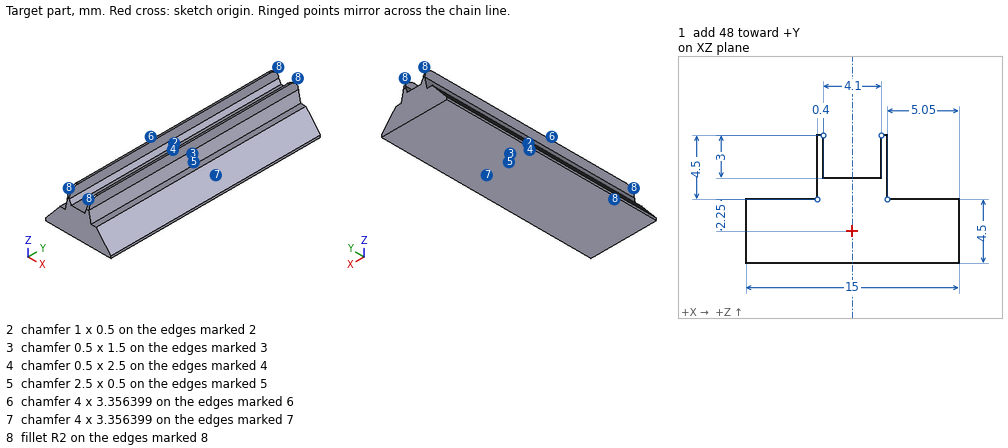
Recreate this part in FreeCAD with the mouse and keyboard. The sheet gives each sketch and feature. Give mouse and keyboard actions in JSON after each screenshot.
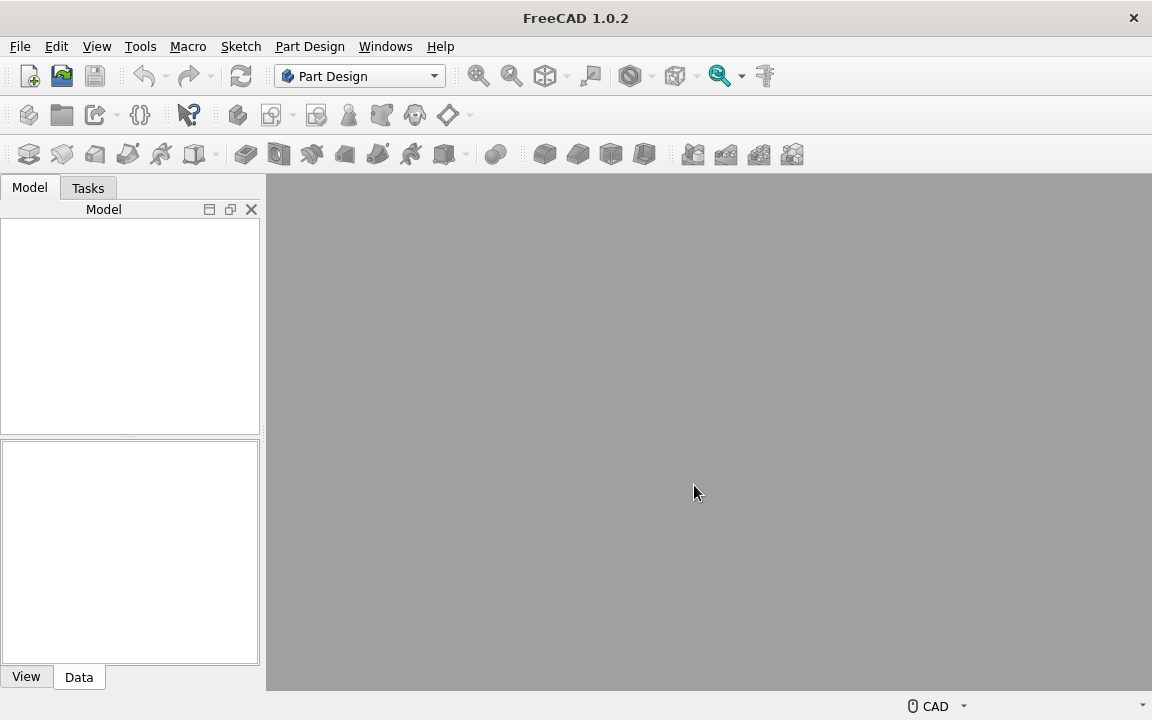
{"action": "left_click", "coordinate": [29, 76]}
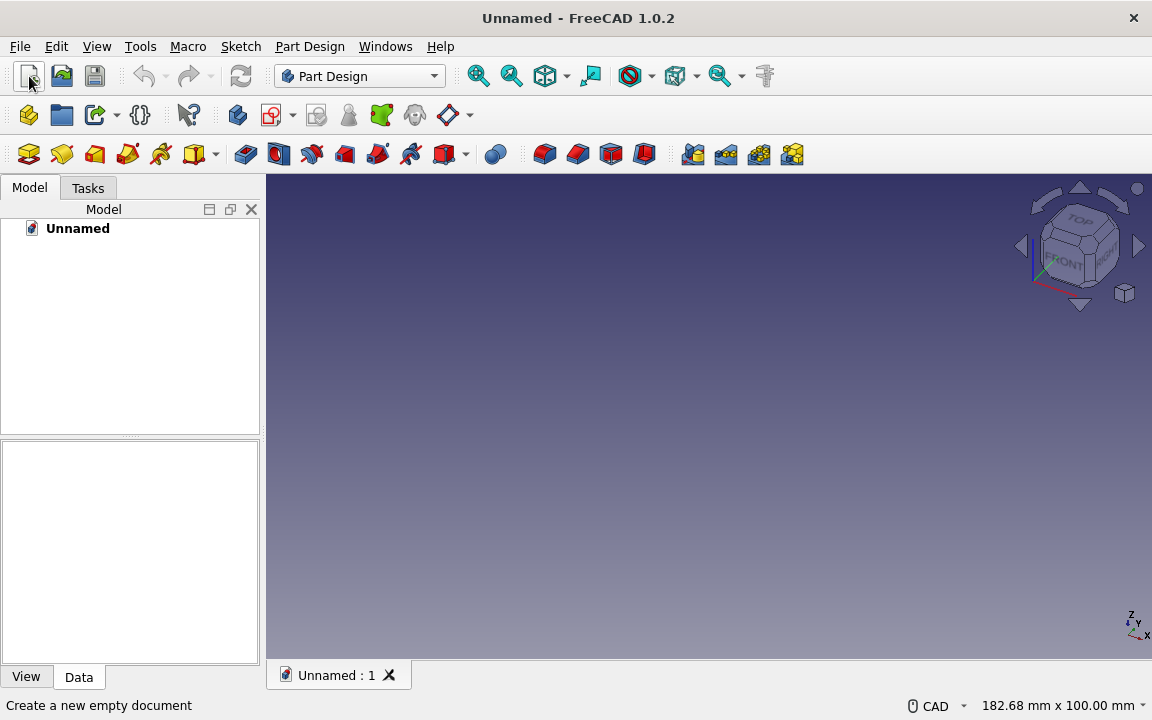
{"action": "left_click", "coordinate": [270, 116]}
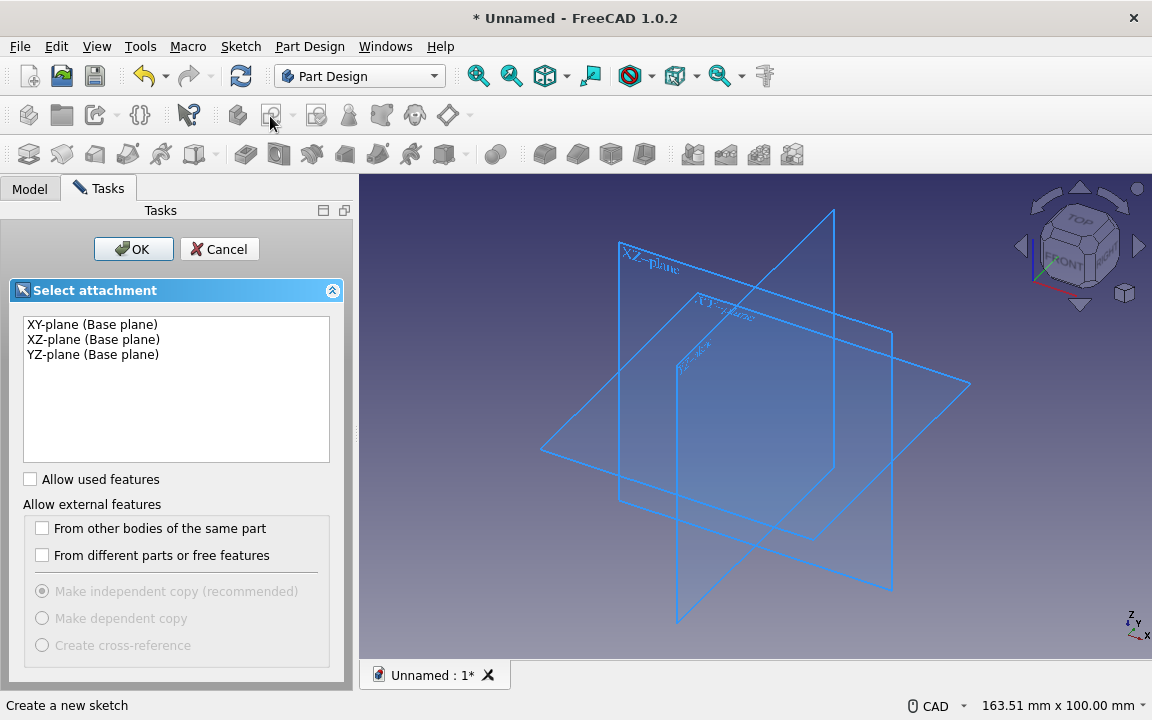
{"action": "left_click", "coordinate": [84, 340]}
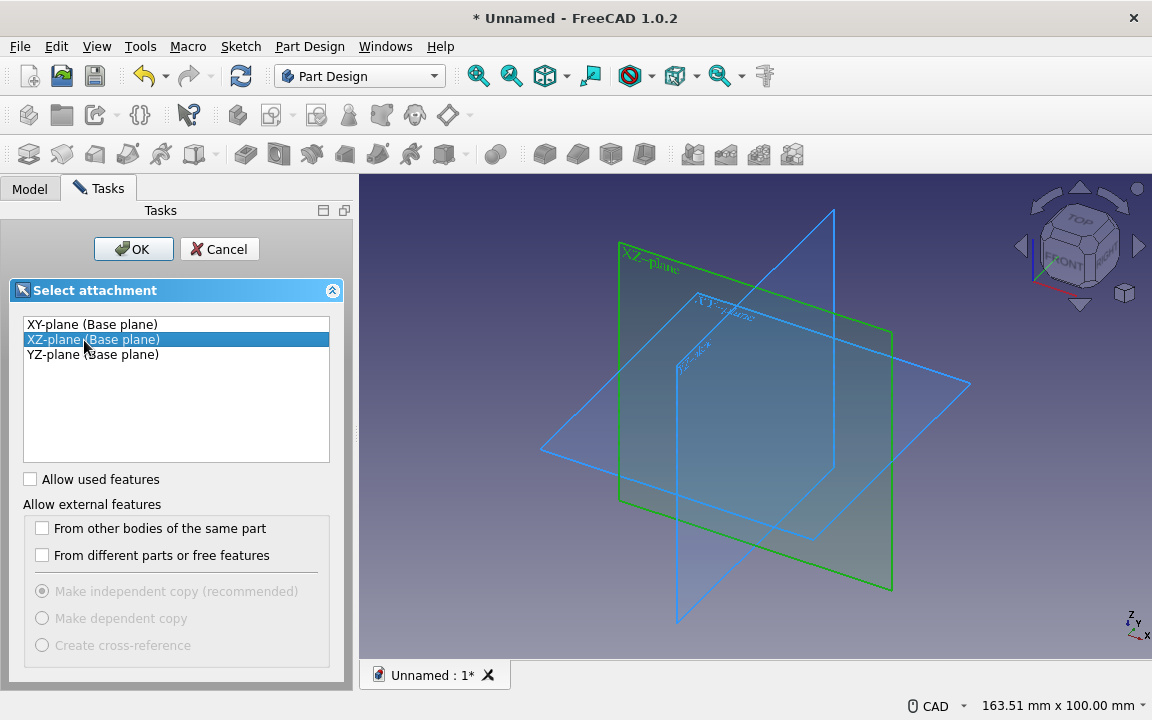
{"action": "left_click", "coordinate": [134, 249]}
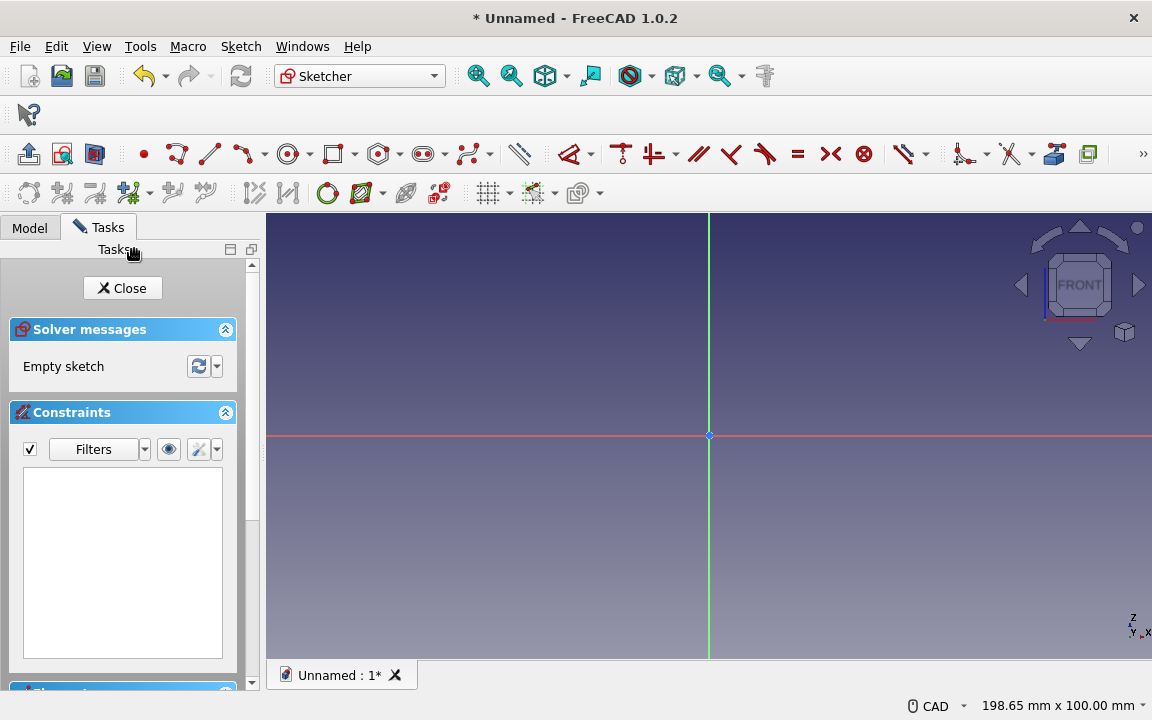
{"action": "scroll", "coordinate": [720, 424], "scroll_direction": "up", "scroll_amount": 10}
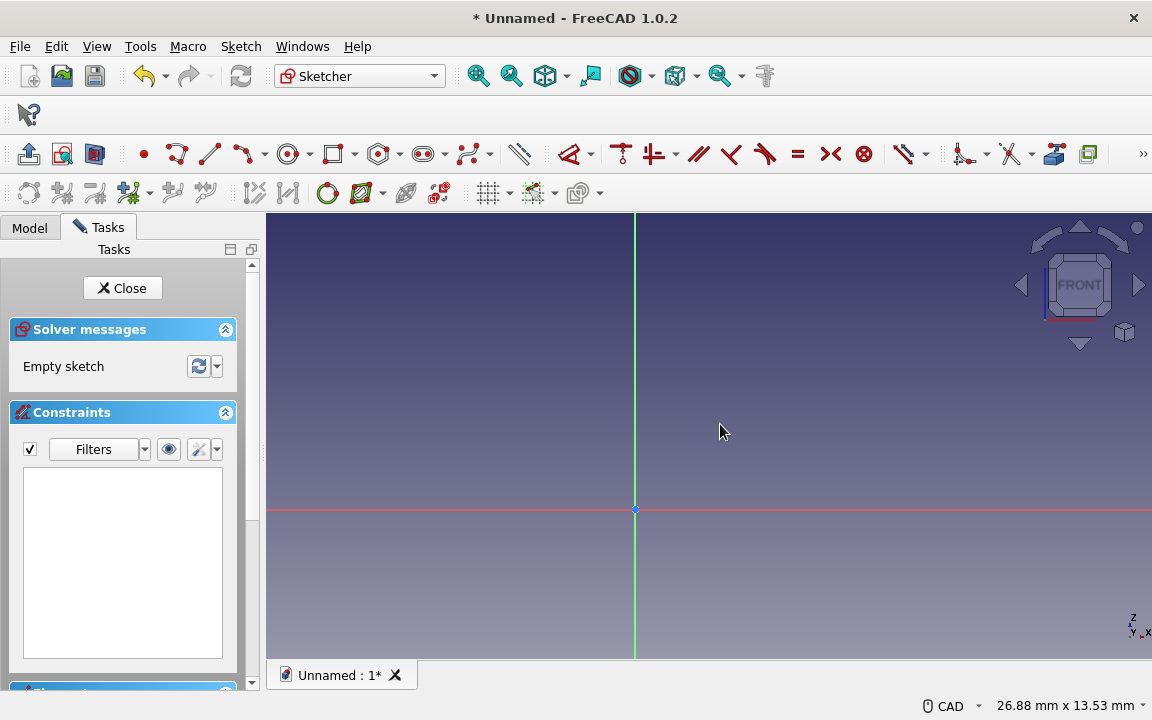
{"action": "left_click", "coordinate": [177, 154]}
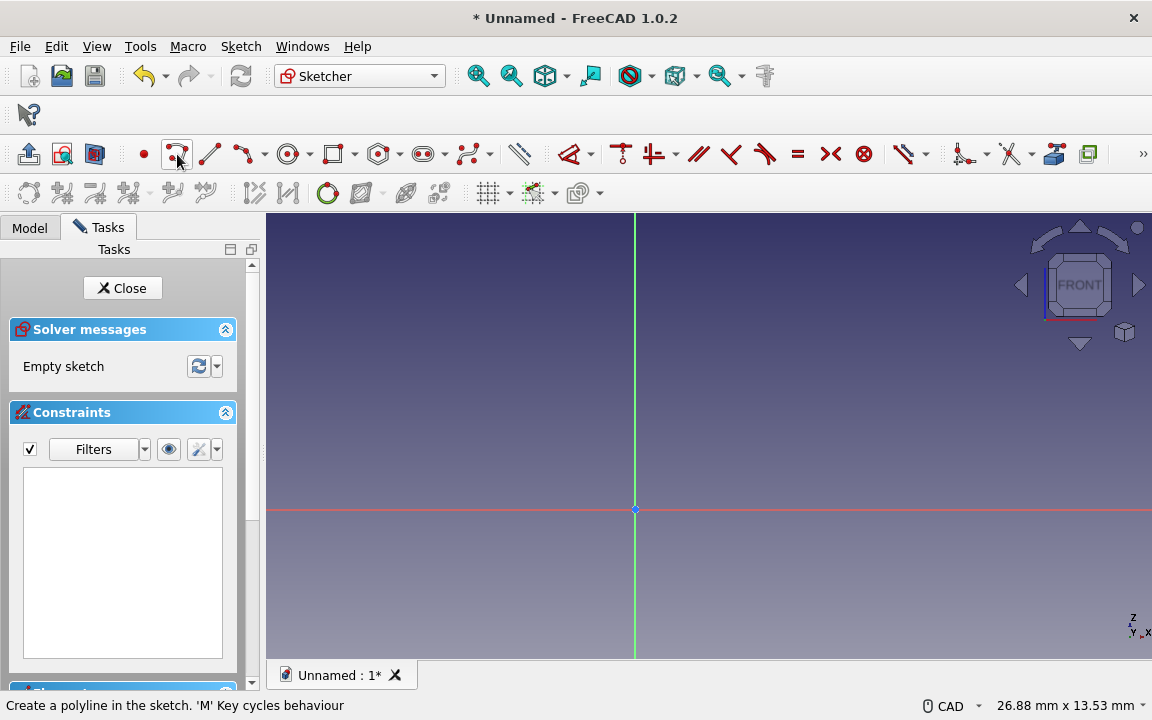
{"action": "left_click", "coordinate": [555, 435]}
{"action": "left_click", "coordinate": [555, 287]}
{"action": "left_click", "coordinate": [568, 287]}
{"action": "left_click", "coordinate": [568, 386]}
{"action": "left_click", "coordinate": [703, 386]}
{"action": "left_click", "coordinate": [703, 287]}
{"action": "left_click", "coordinate": [716, 287]}
{"action": "left_click", "coordinate": [716, 435]}
{"action": "left_click", "coordinate": [883, 435]}
{"action": "left_click", "coordinate": [883, 584]}
{"action": "left_click", "coordinate": [388, 584]}
{"action": "left_click", "coordinate": [388, 435]}
{"action": "left_click", "coordinate": [555, 436]}
{"action": "key", "text": "Escape"}
{"action": "key", "text": "Escape"}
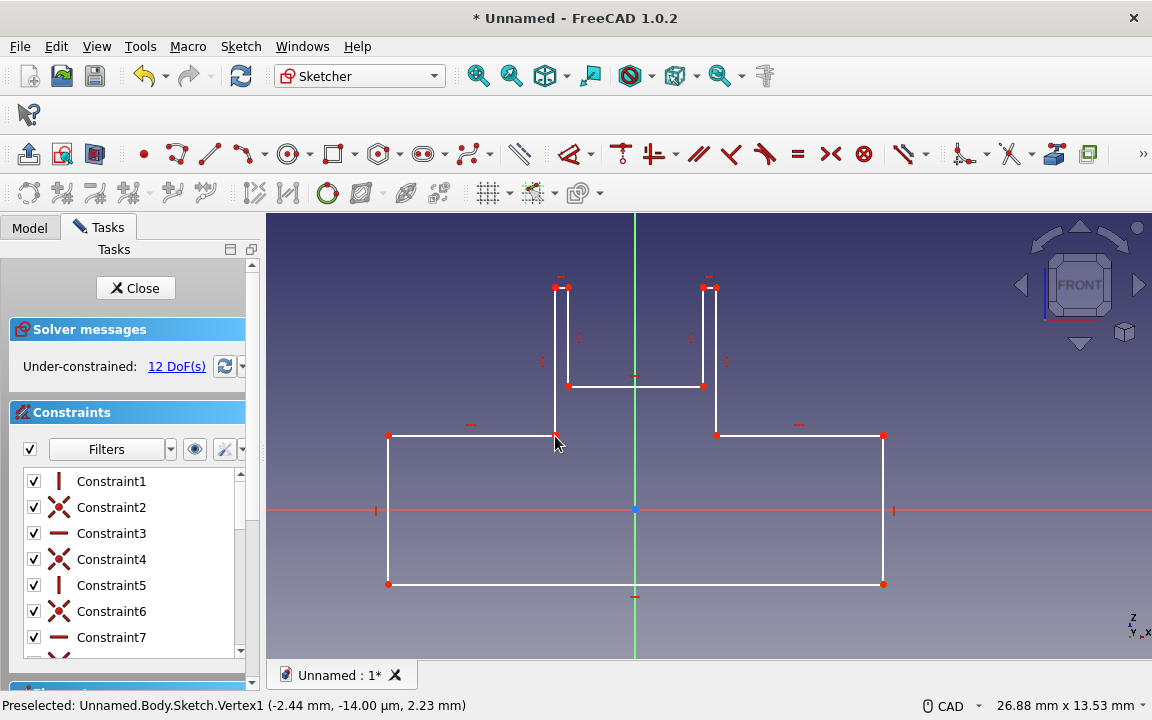
{"action": "left_click", "coordinate": [568, 288]}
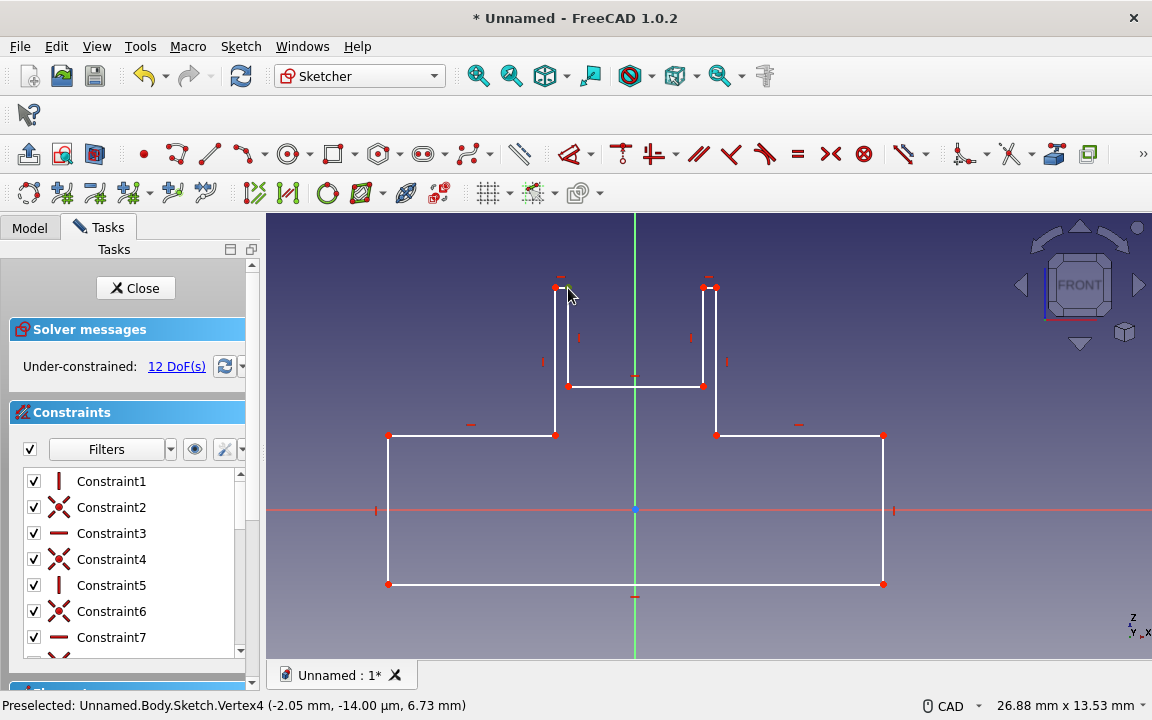
{"action": "left_click", "coordinate": [703, 288]}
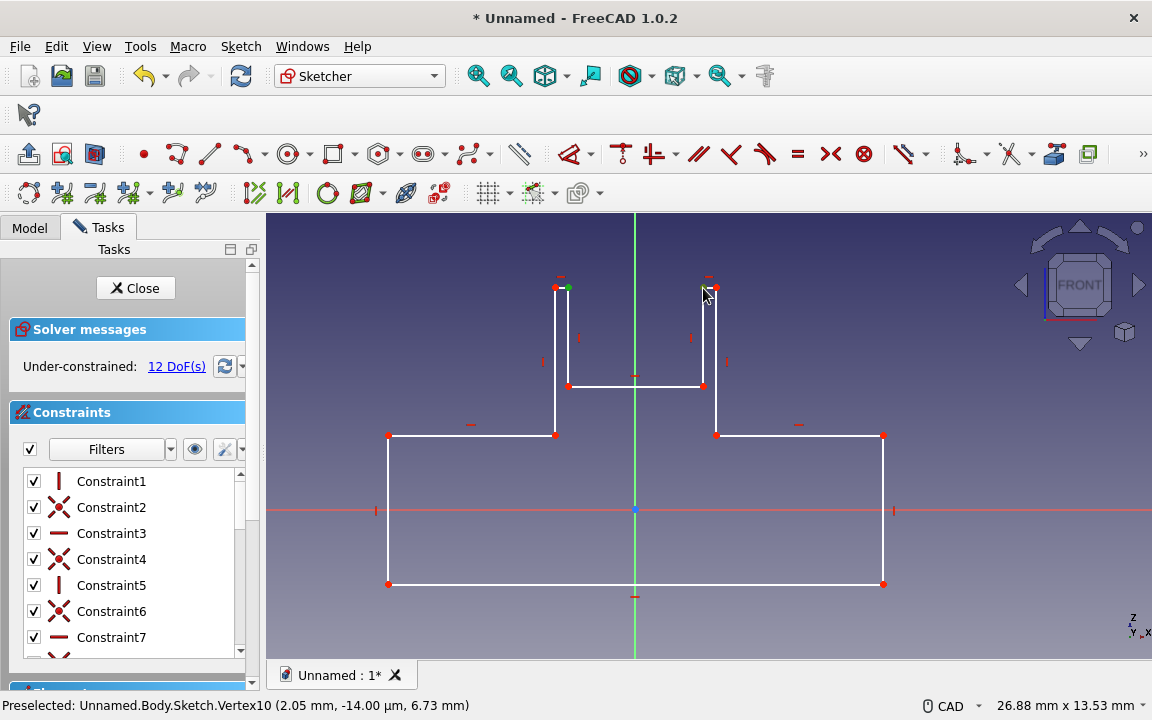
{"action": "left_click", "coordinate": [635, 547]}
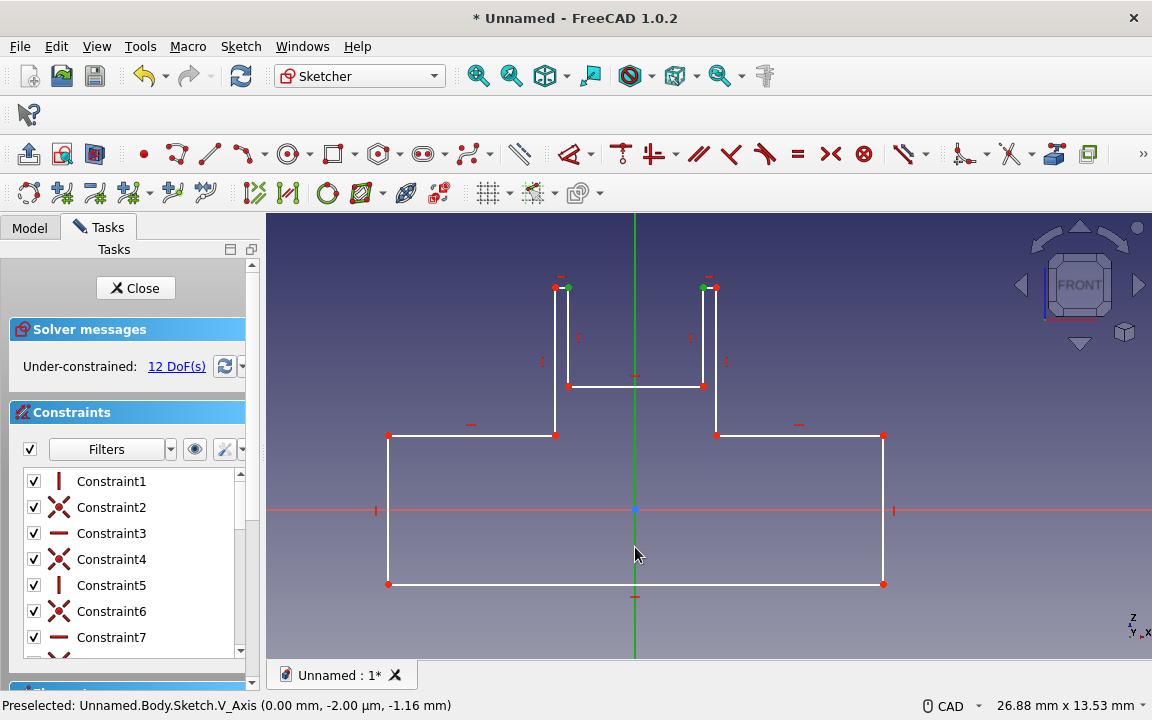
{"action": "key", "text": "s"}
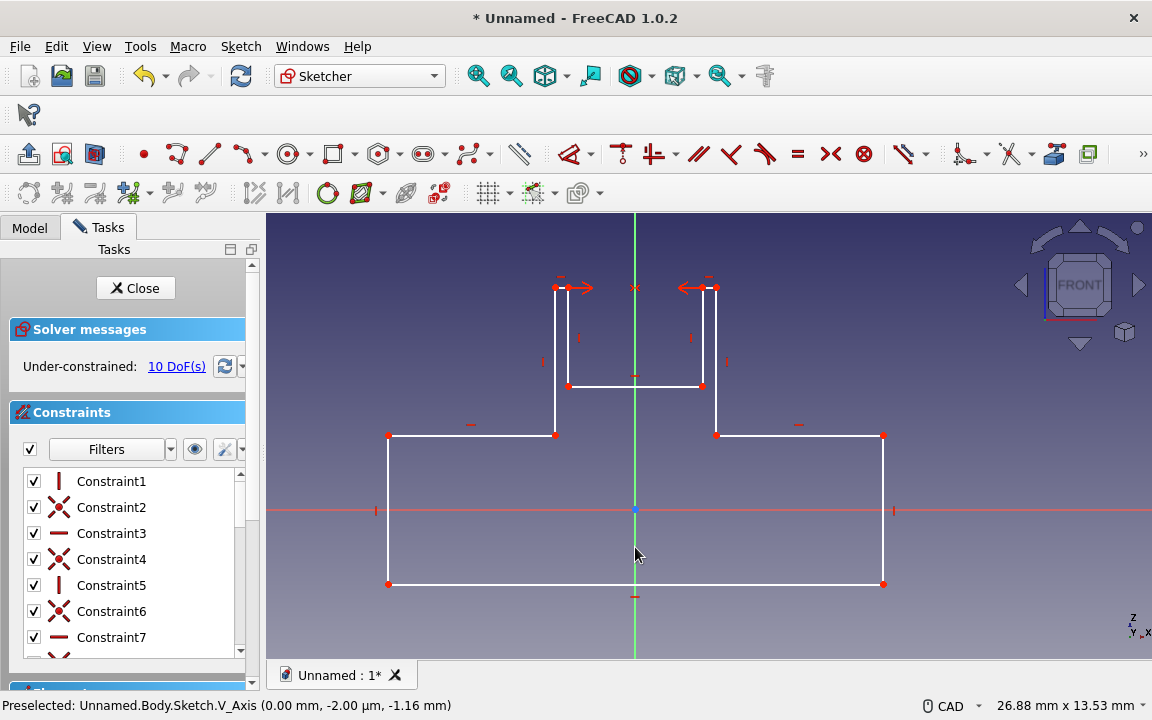
{"action": "left_click", "coordinate": [555, 436]}